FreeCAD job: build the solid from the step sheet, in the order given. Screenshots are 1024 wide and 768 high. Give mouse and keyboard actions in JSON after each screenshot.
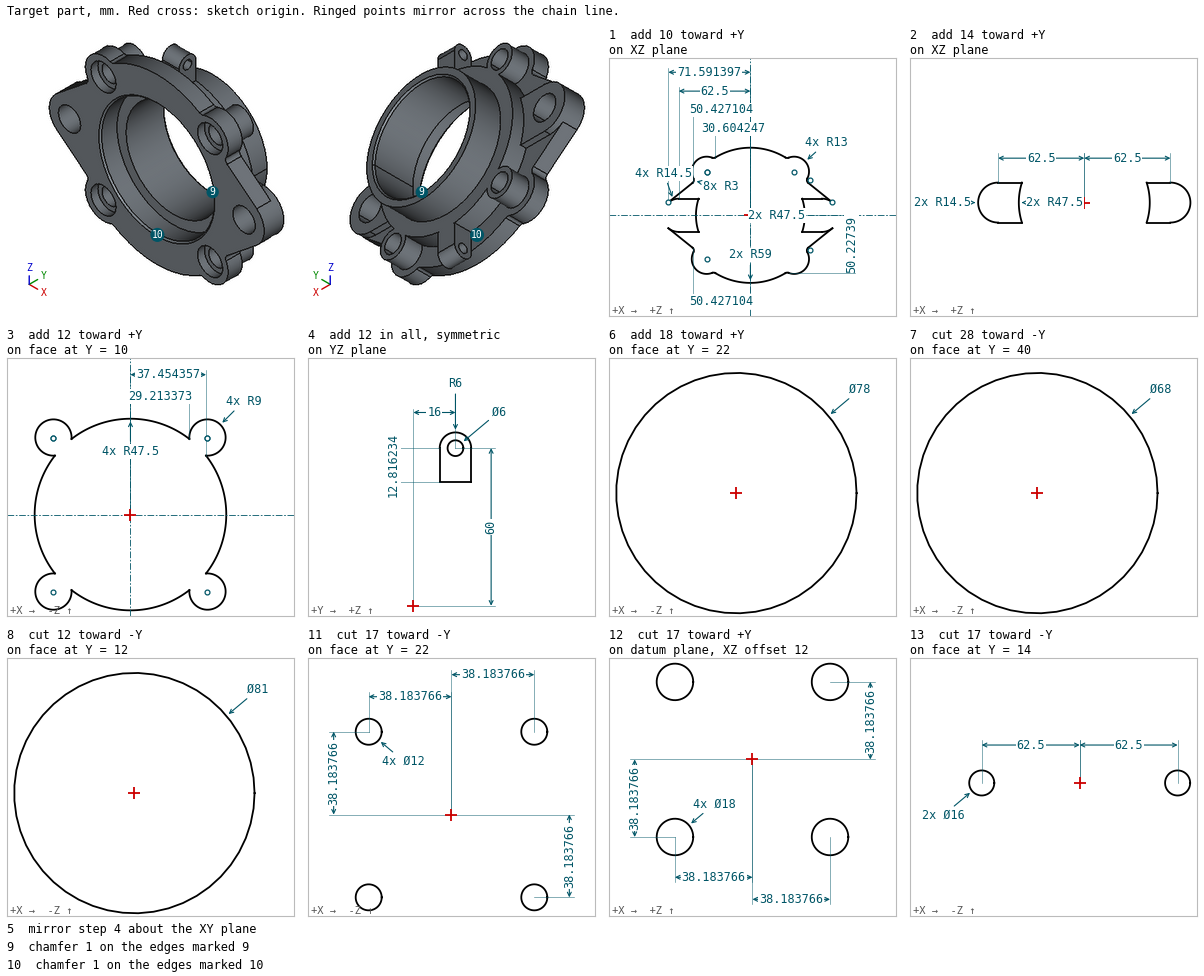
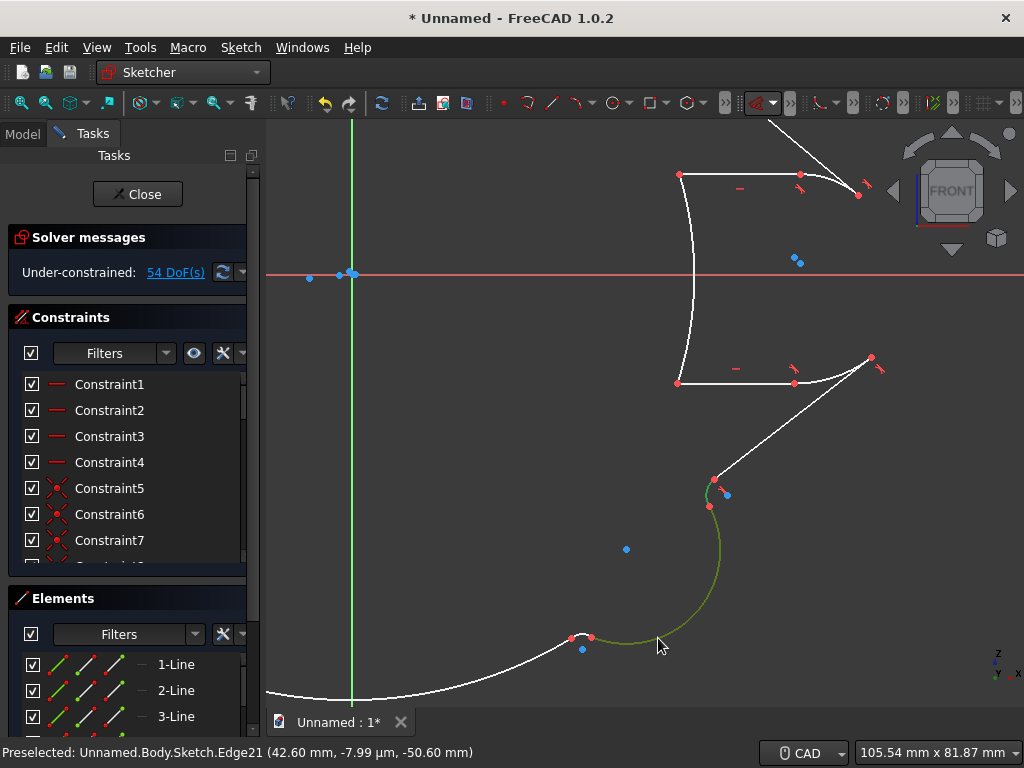
{"action": "key", "text": "t"}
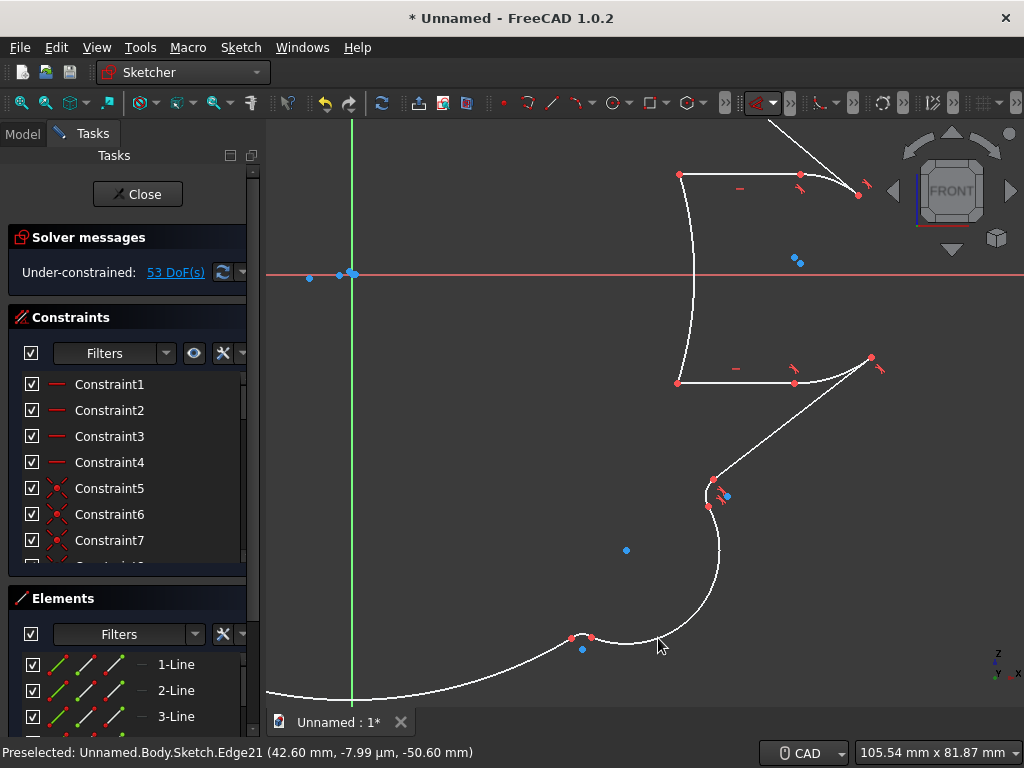
{"action": "left_click", "coordinate": [658, 638]}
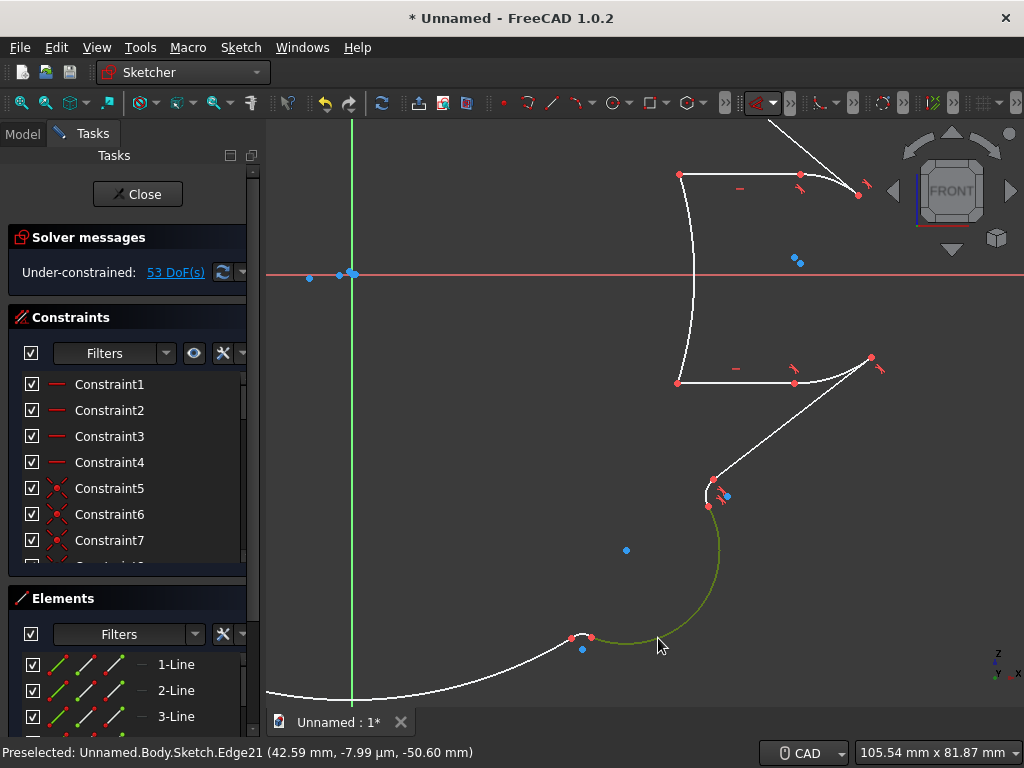
{"action": "scroll", "coordinate": [581, 634], "scroll_direction": "up", "scroll_amount": 2}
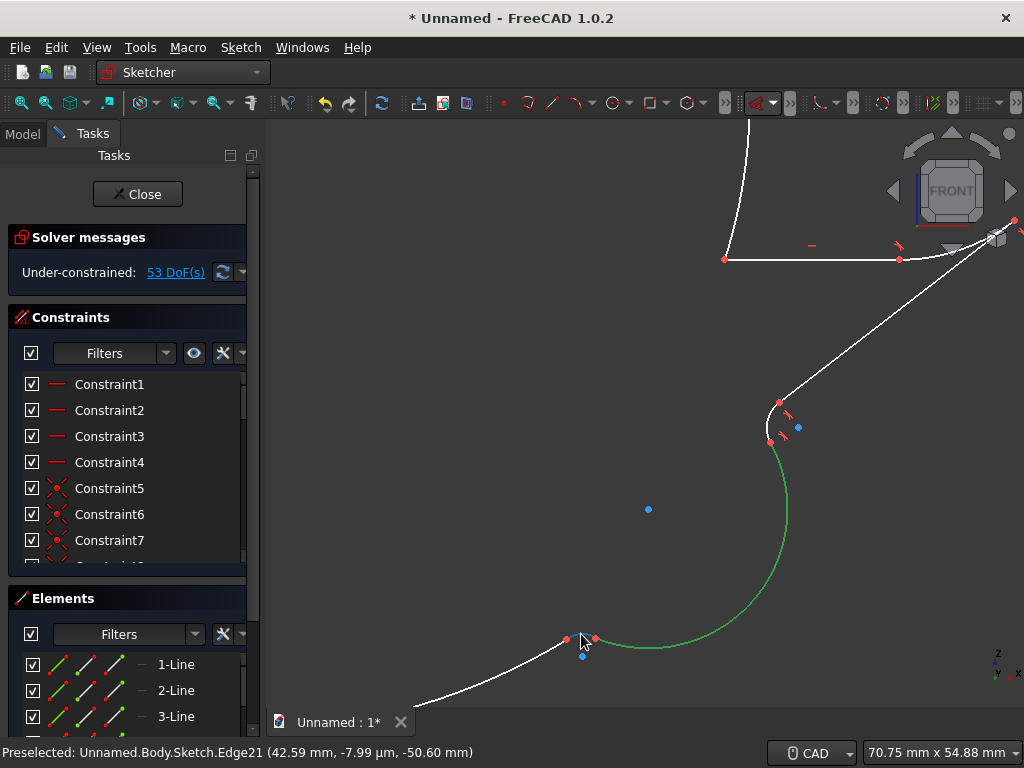
{"action": "left_click", "coordinate": [581, 634]}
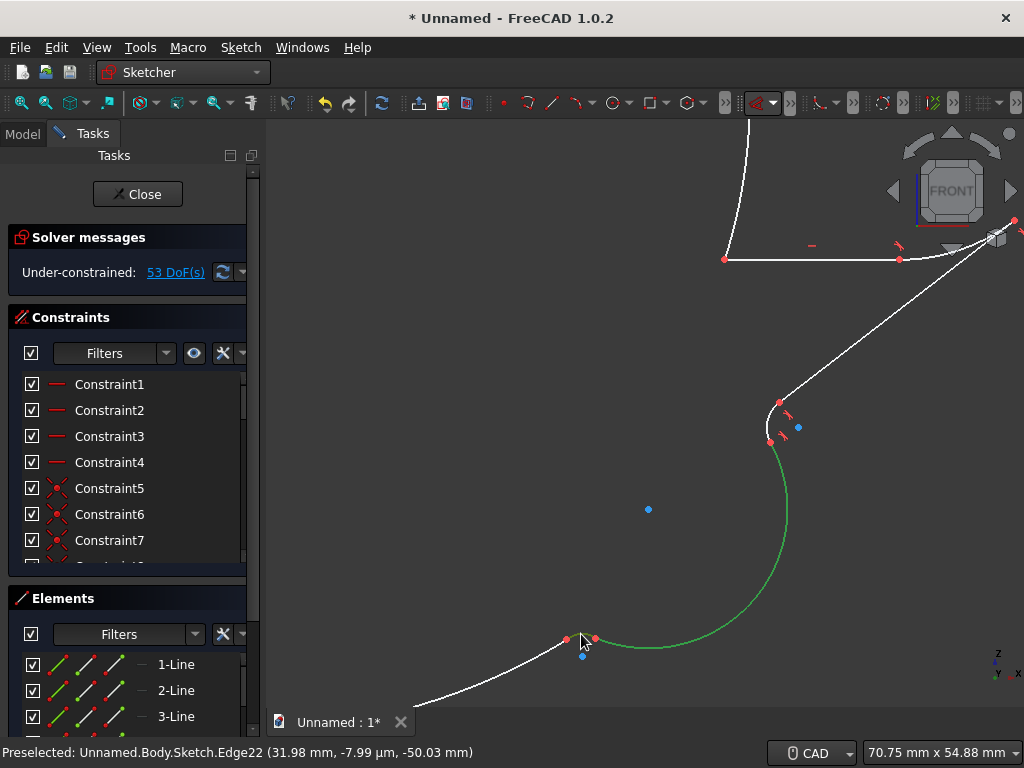
{"action": "key", "text": "t"}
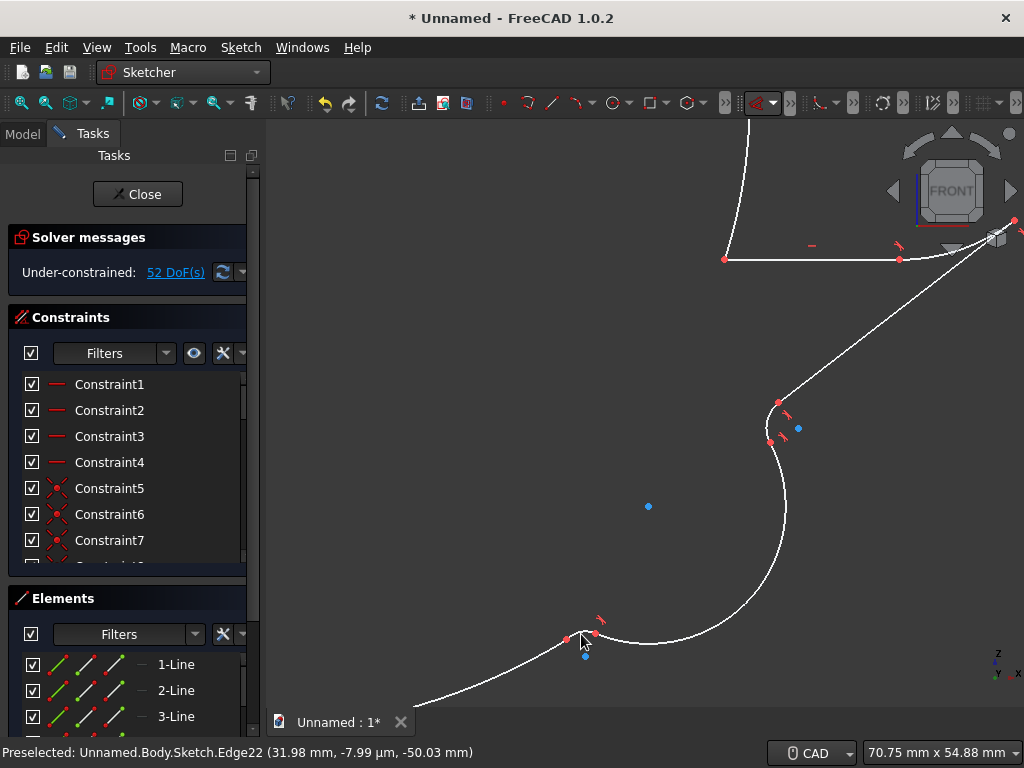
{"action": "scroll", "coordinate": [586, 631], "scroll_direction": "up", "scroll_amount": 2}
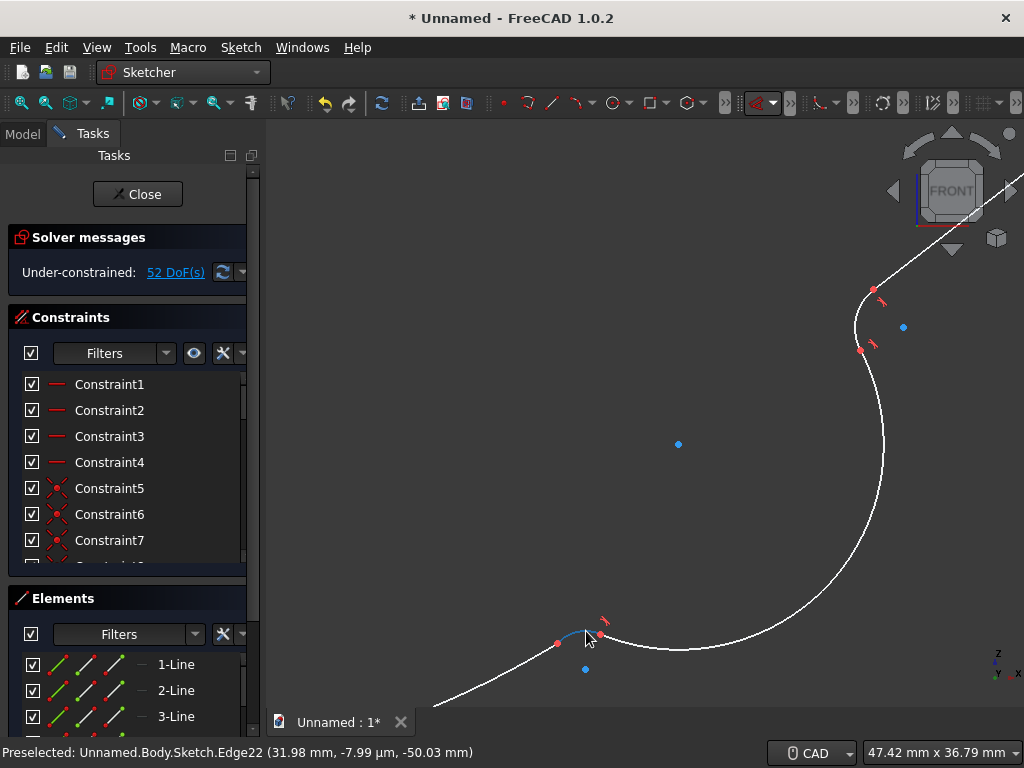
{"action": "left_click", "coordinate": [586, 631]}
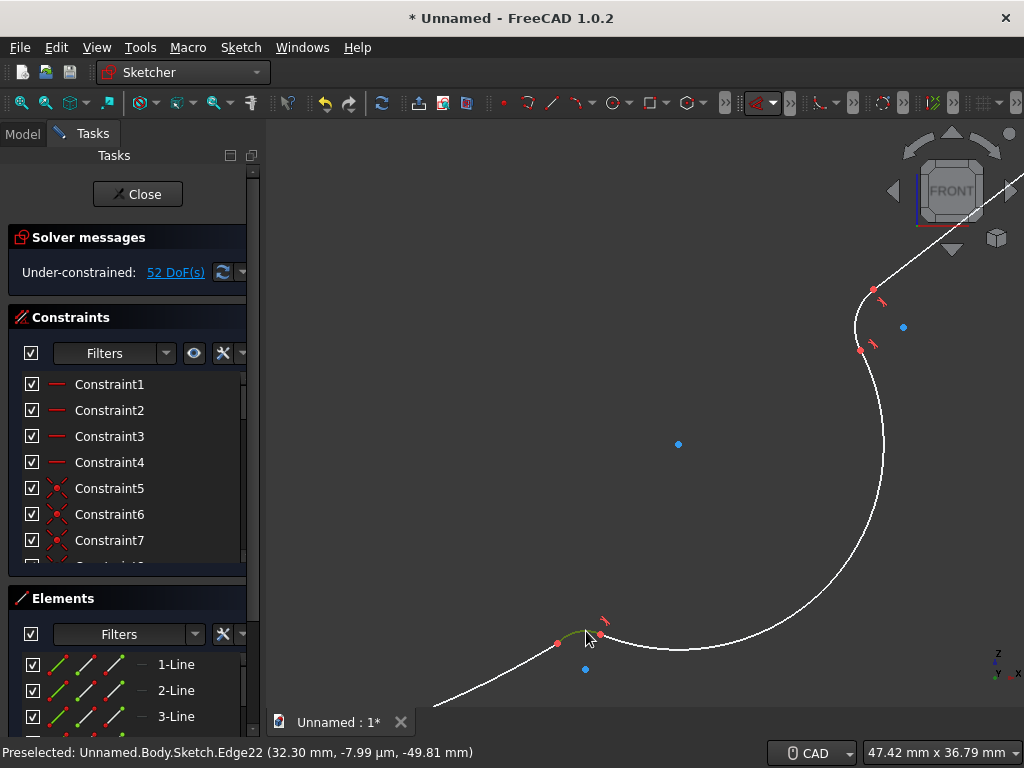
{"action": "scroll", "coordinate": [677, 527], "scroll_direction": "down", "scroll_amount": 9}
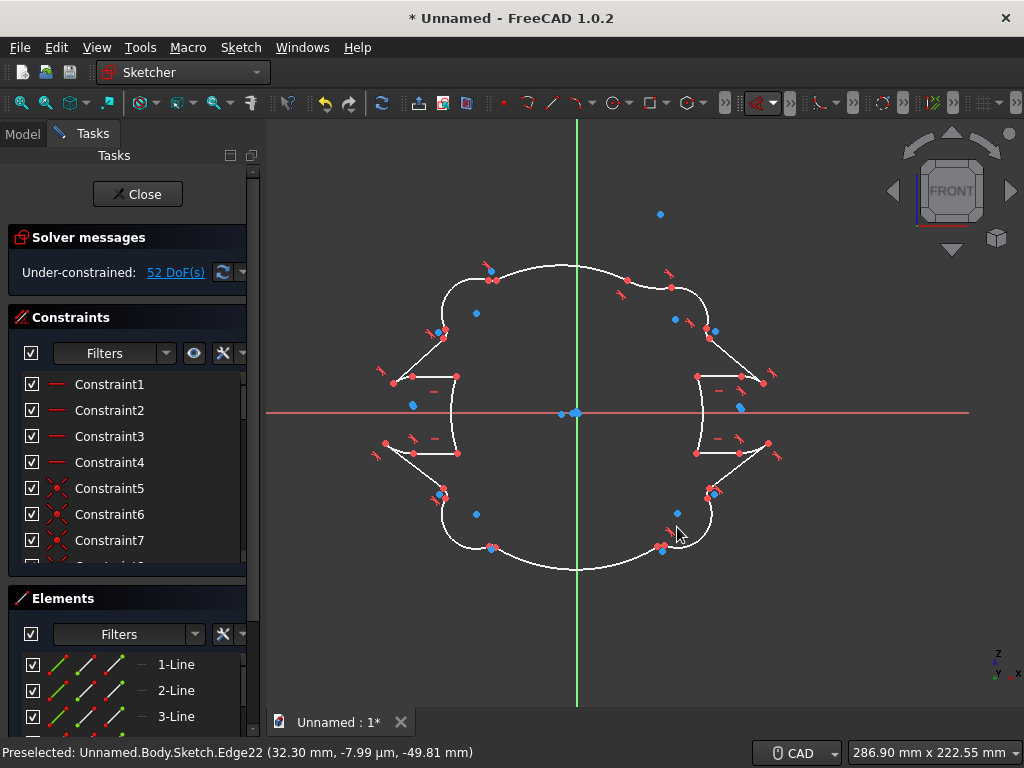
{"action": "left_click", "coordinate": [543, 566]}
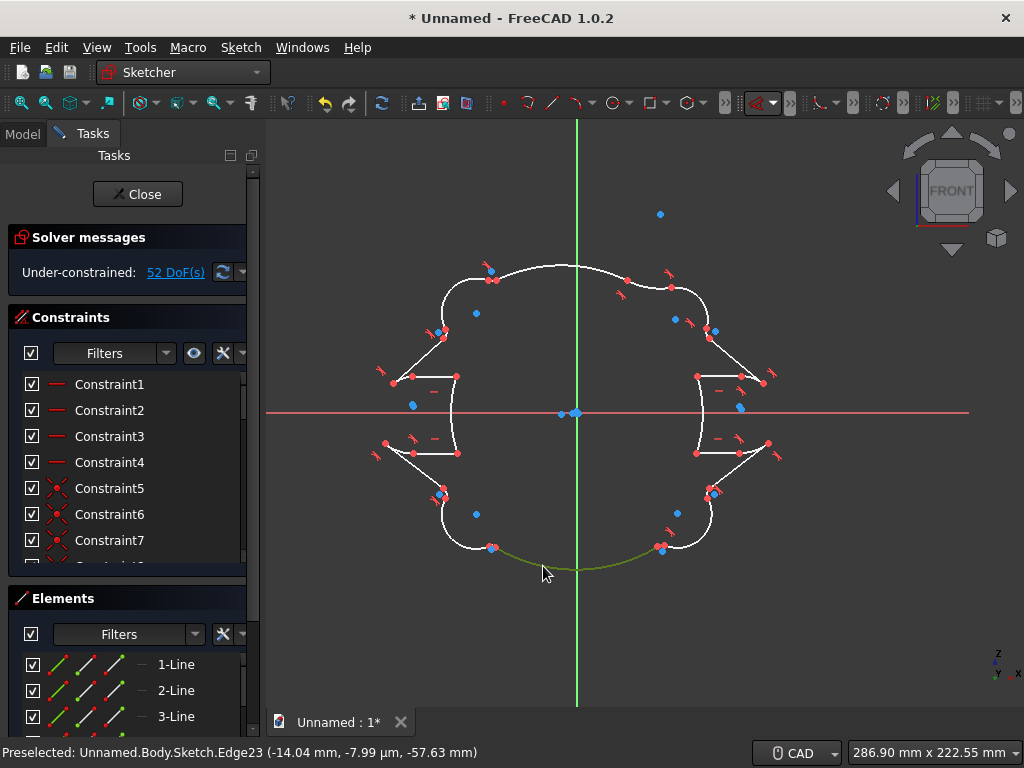
{"action": "key", "text": "t"}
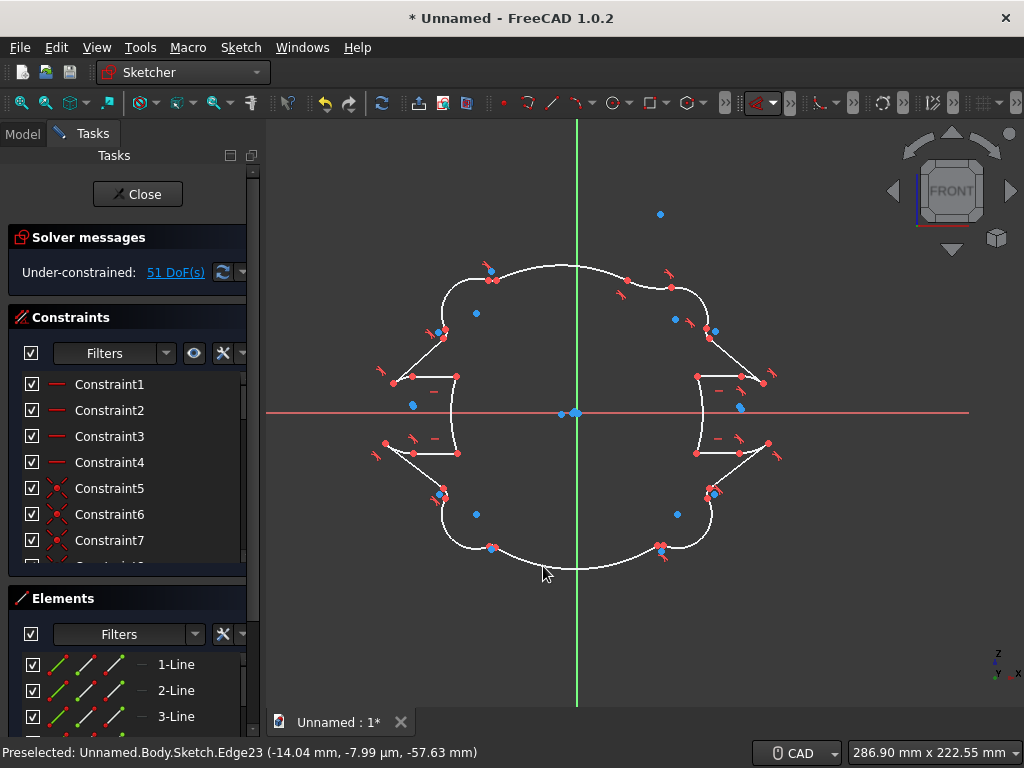
{"action": "left_click", "coordinate": [543, 566]}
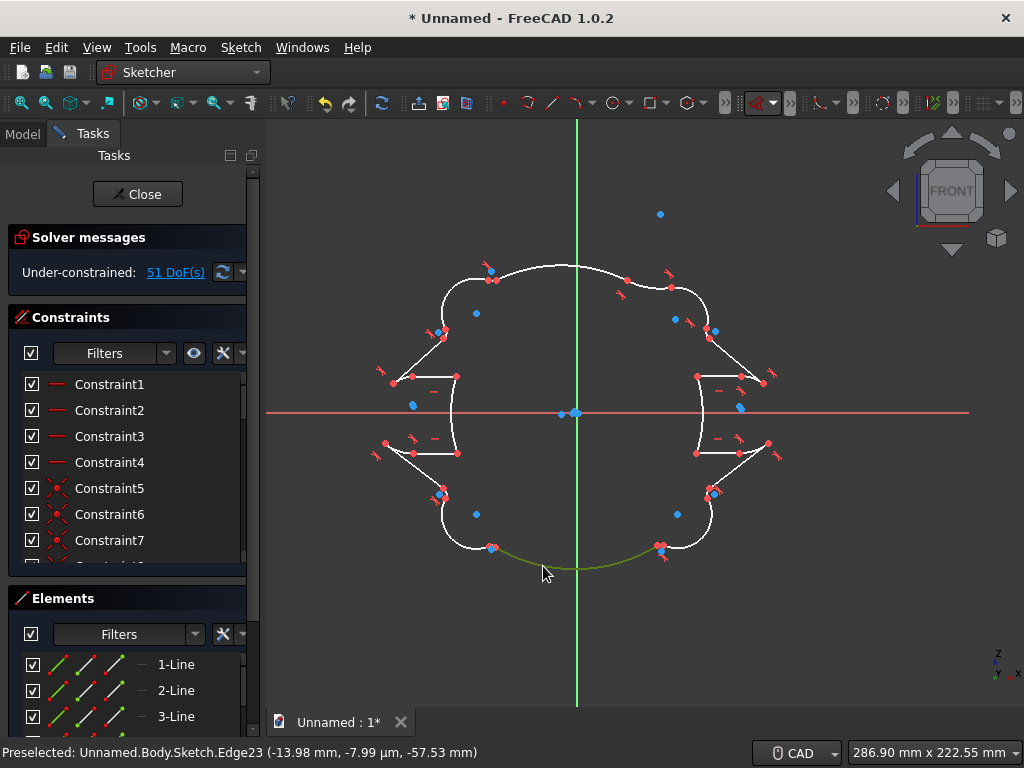
{"action": "scroll", "coordinate": [493, 545], "scroll_direction": "up", "scroll_amount": 7}